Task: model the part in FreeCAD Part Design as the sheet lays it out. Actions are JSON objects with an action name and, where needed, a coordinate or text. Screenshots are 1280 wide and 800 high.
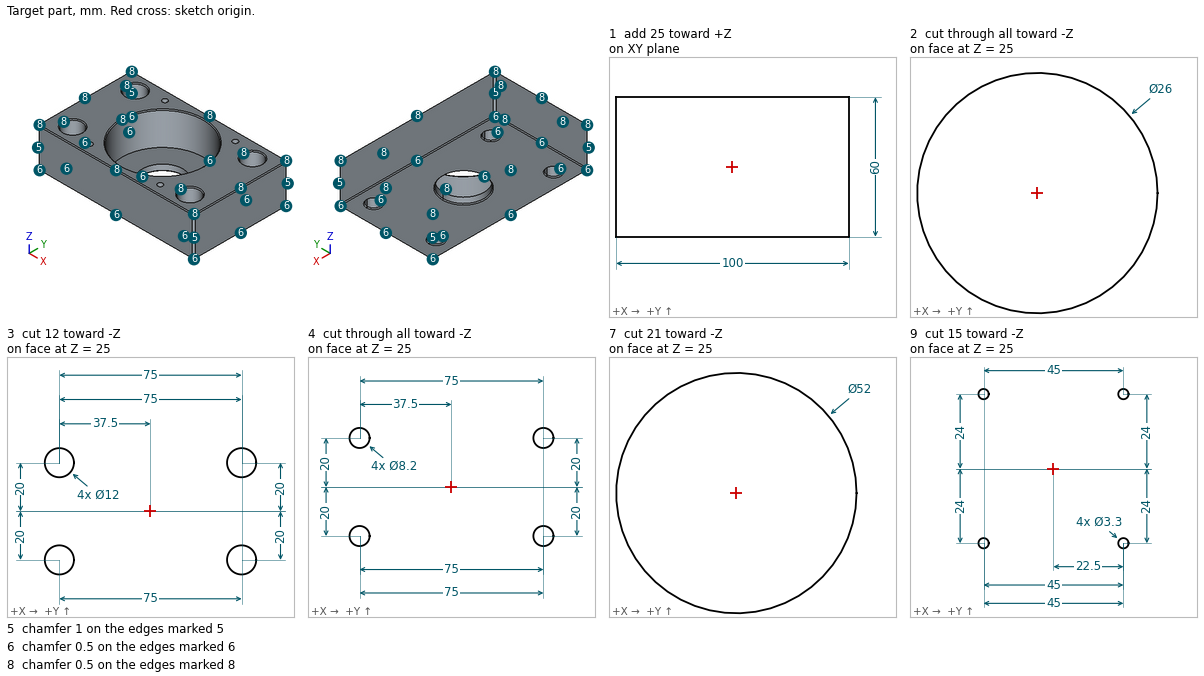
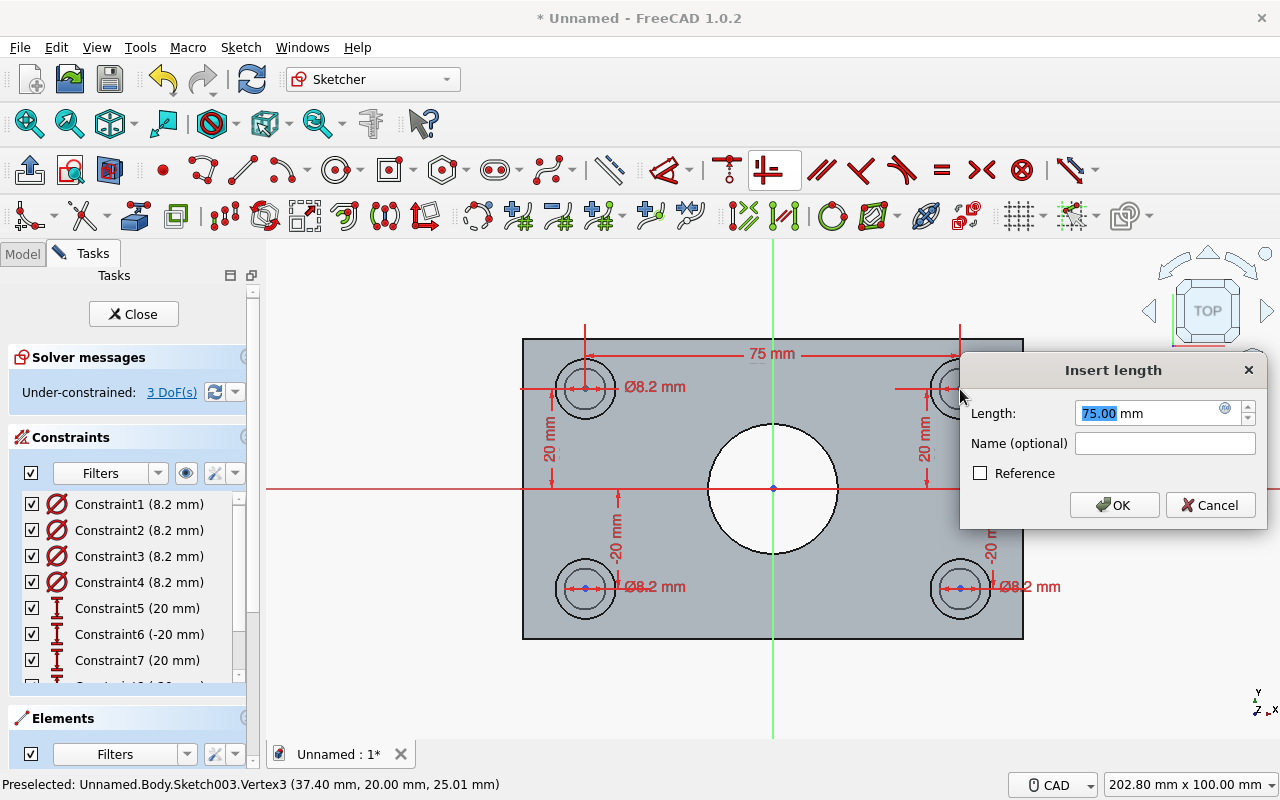
{"action": "type", "text": "75"}
{"action": "key", "text": "Return"}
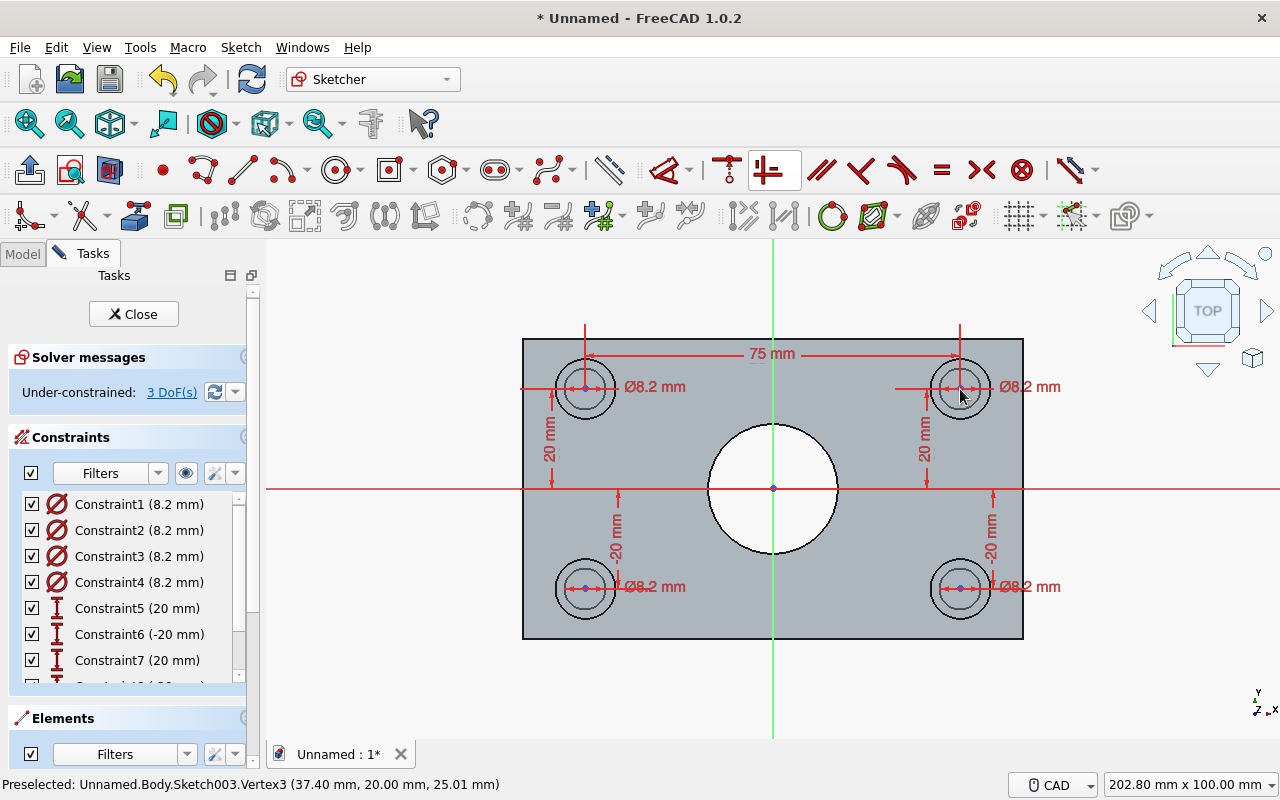
{"action": "left_click", "coordinate": [585, 589]}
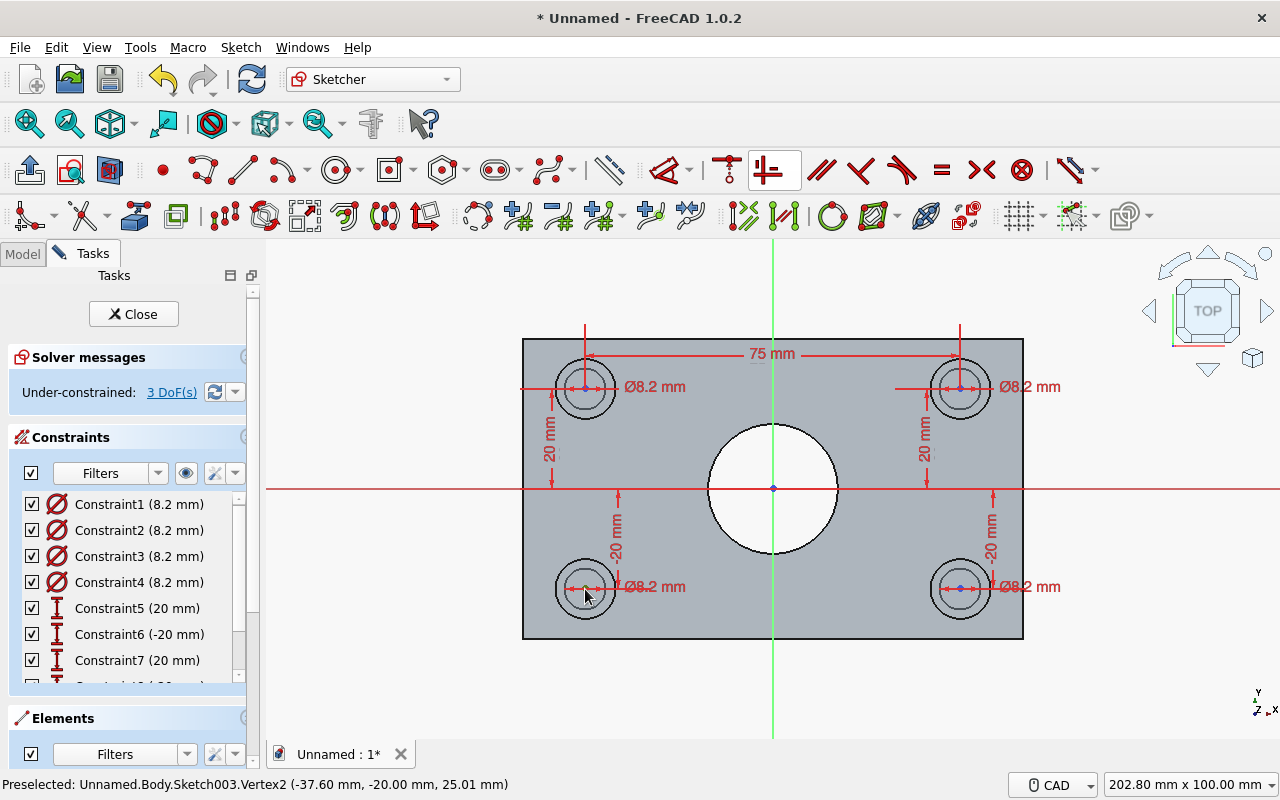
{"action": "left_click", "coordinate": [960, 389]}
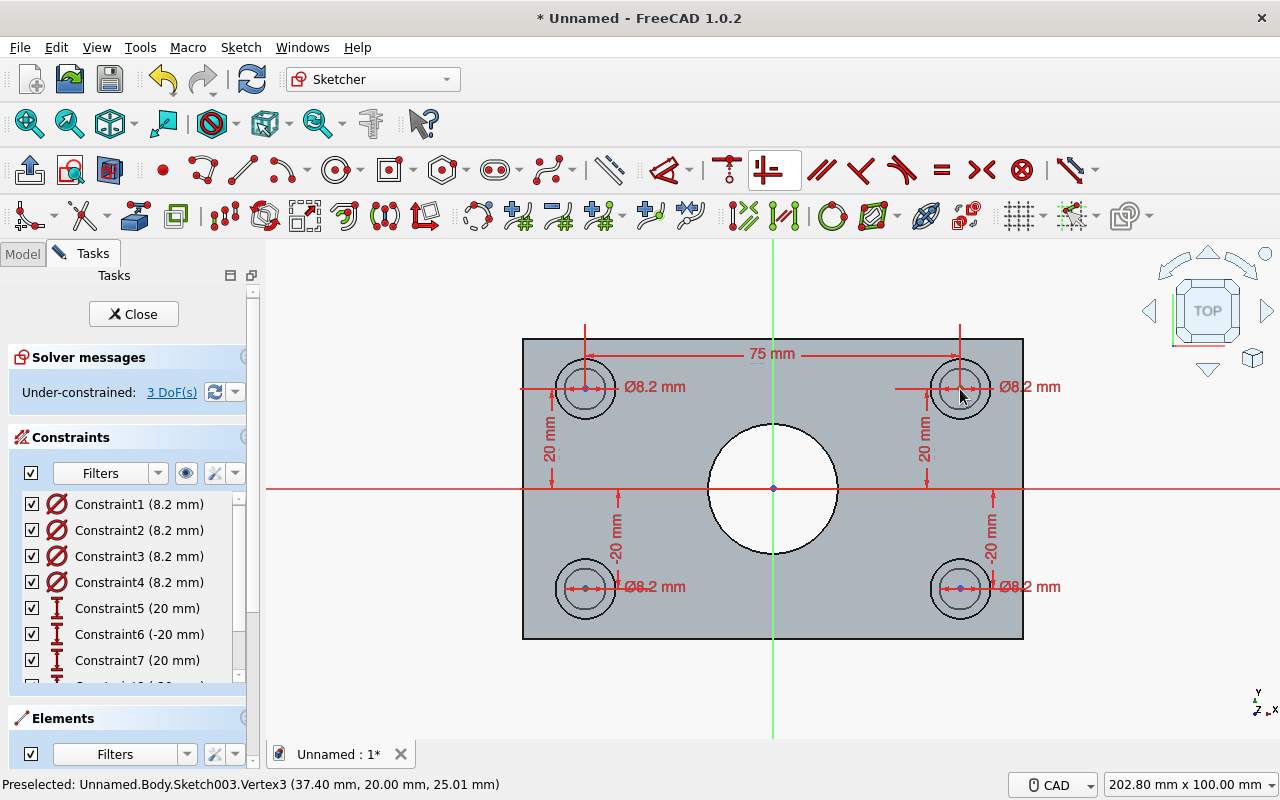
{"action": "key", "text": "l"}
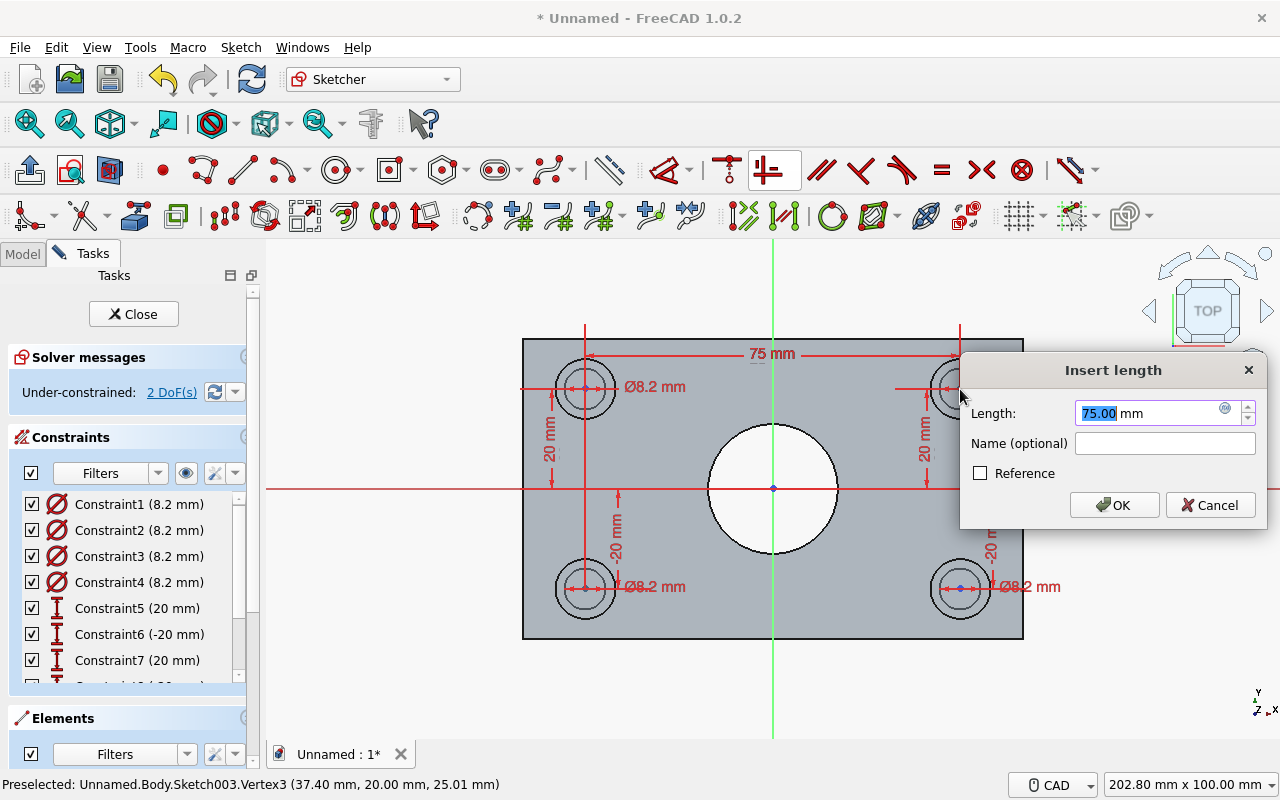
{"action": "type", "text": "75"}
{"action": "key", "text": "Return"}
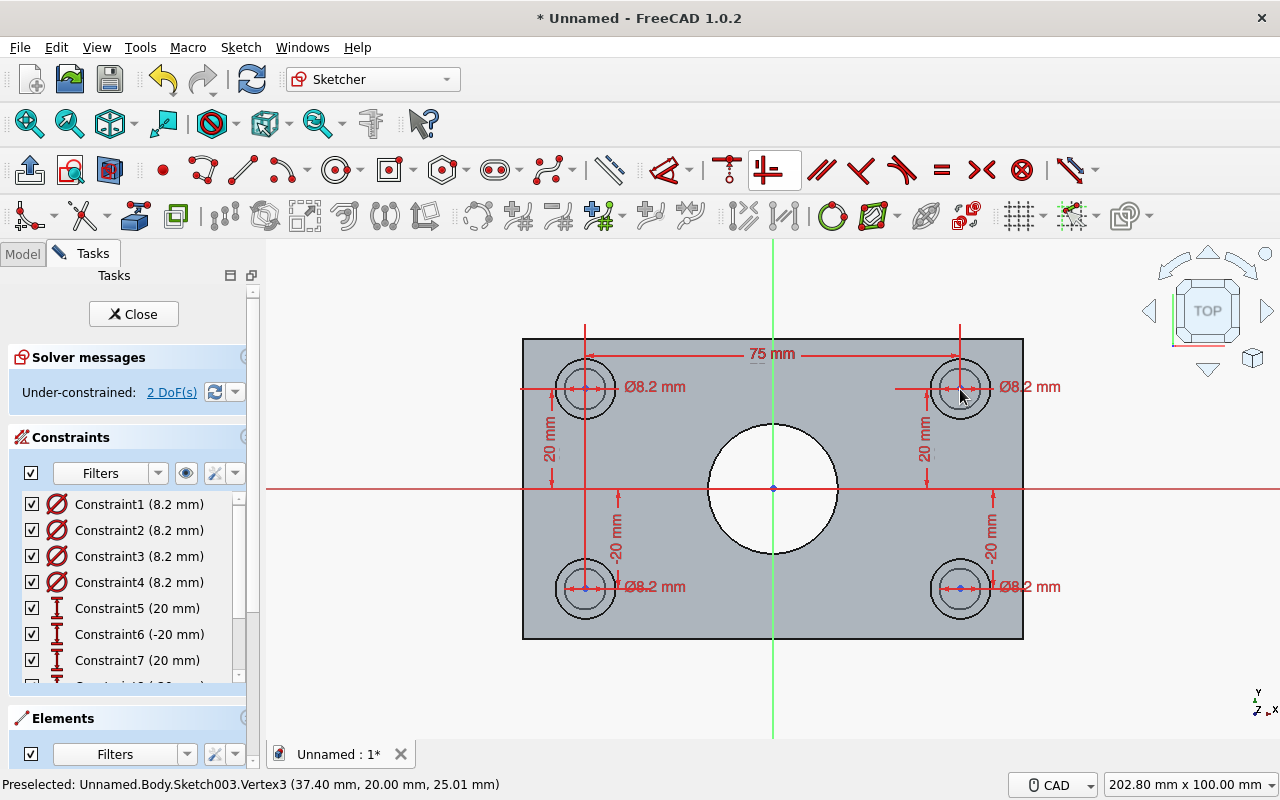
{"action": "left_click", "coordinate": [585, 589]}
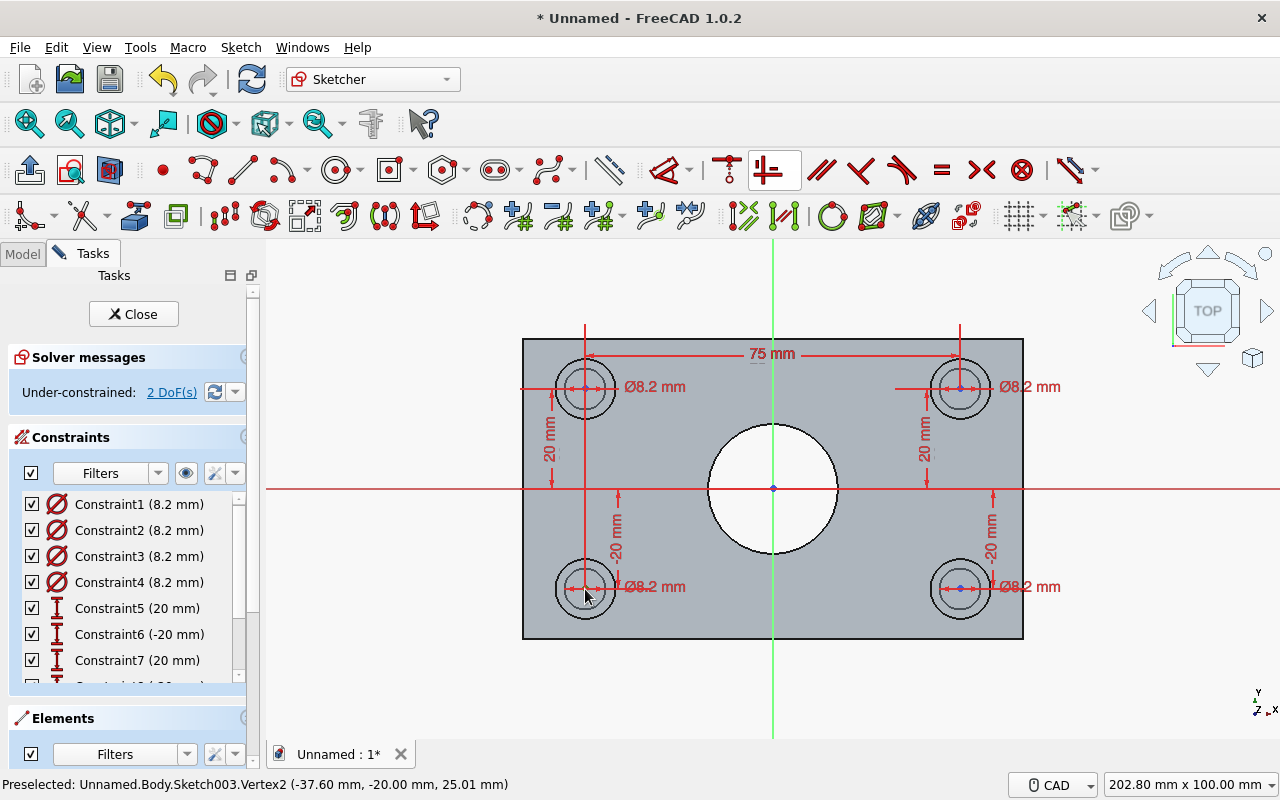
{"action": "left_click", "coordinate": [960, 589]}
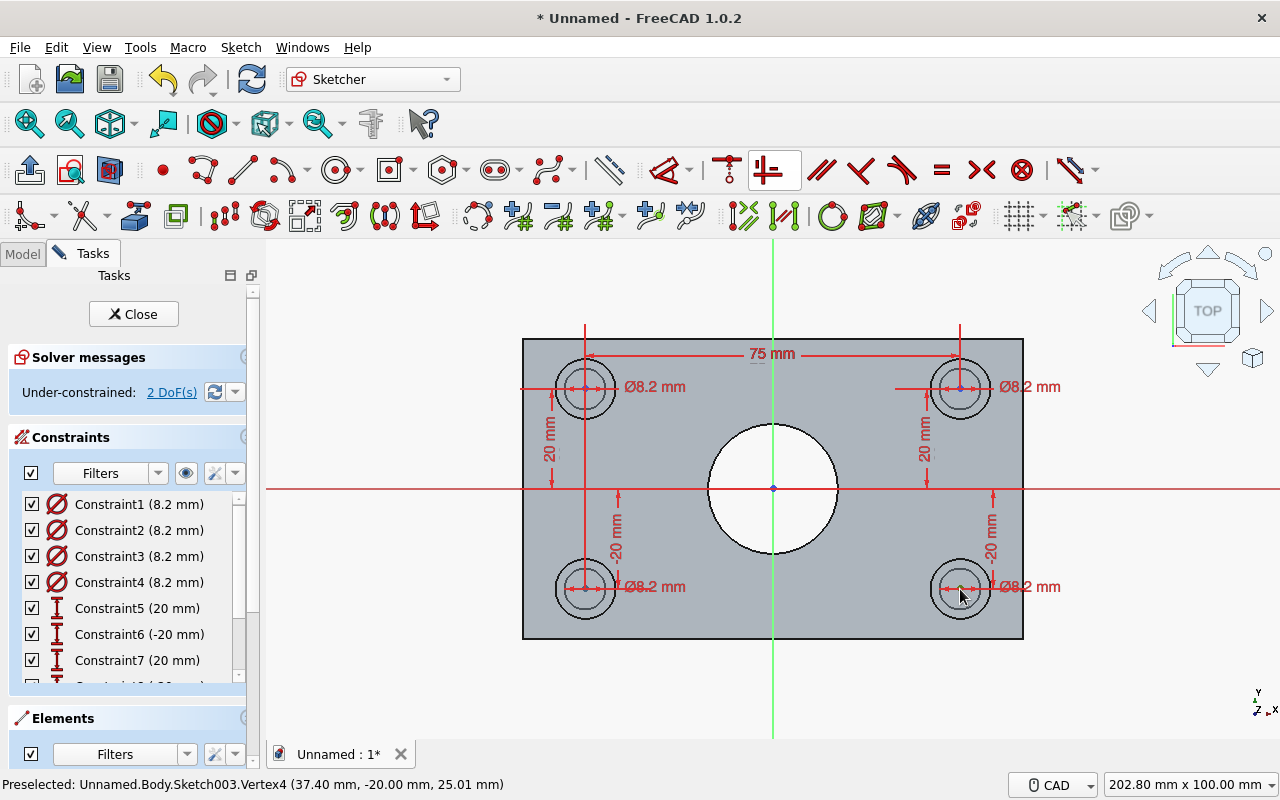
{"action": "left_click", "coordinate": [692, 170]}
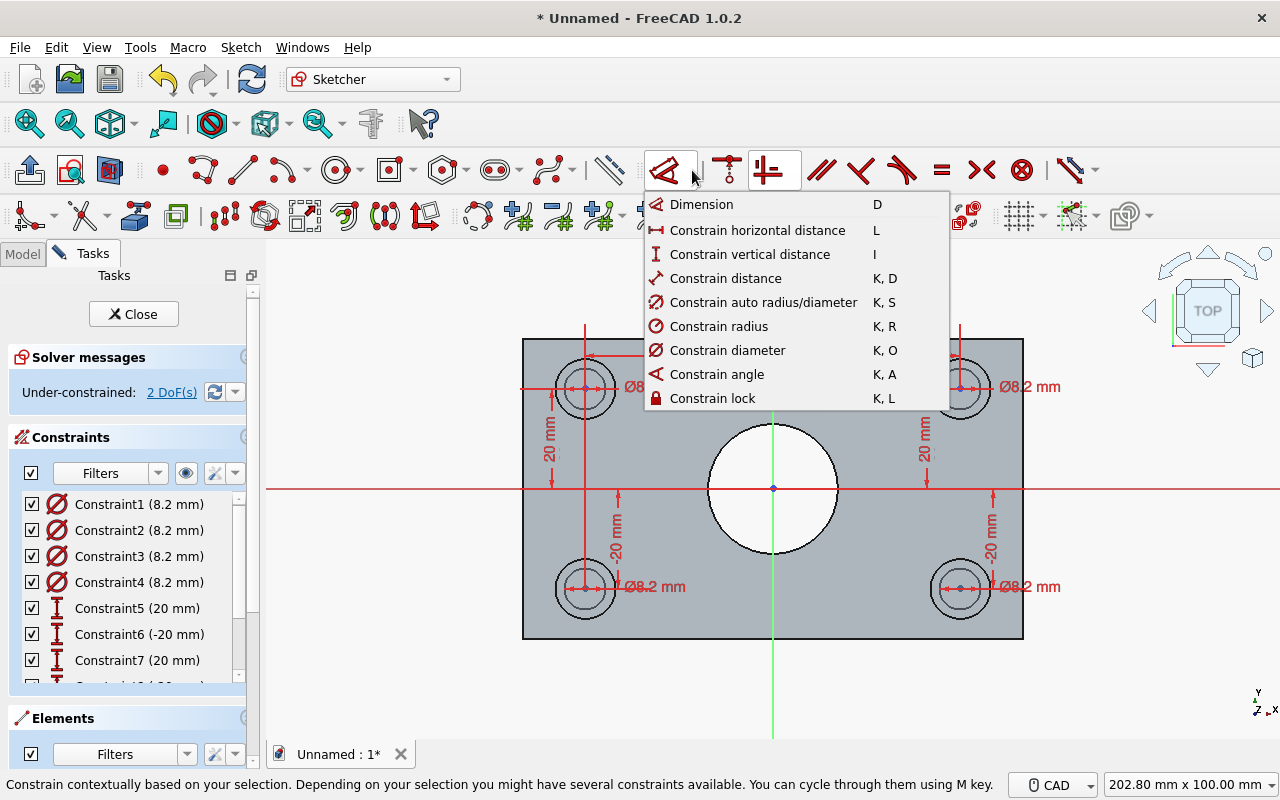
{"action": "left_click", "coordinate": [797, 230]}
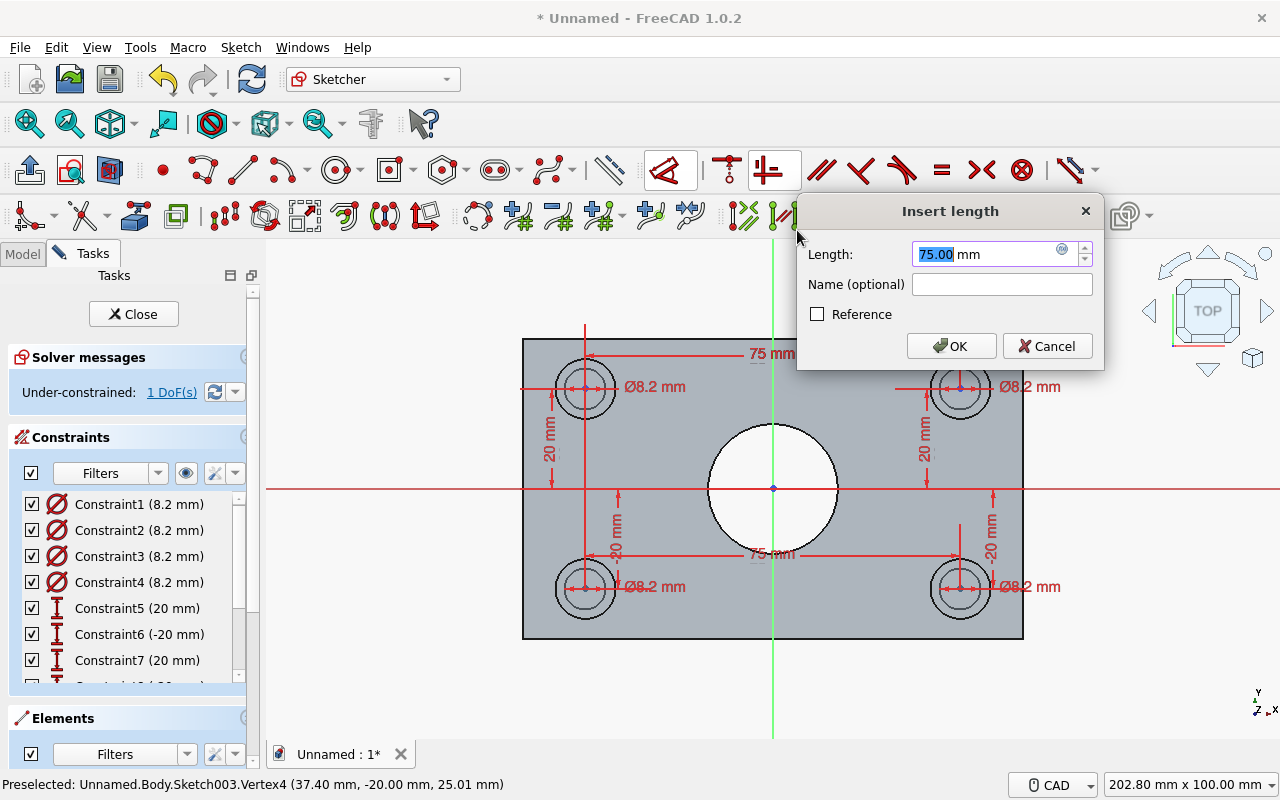
{"action": "type", "text": "75"}
{"action": "key", "text": "Return"}